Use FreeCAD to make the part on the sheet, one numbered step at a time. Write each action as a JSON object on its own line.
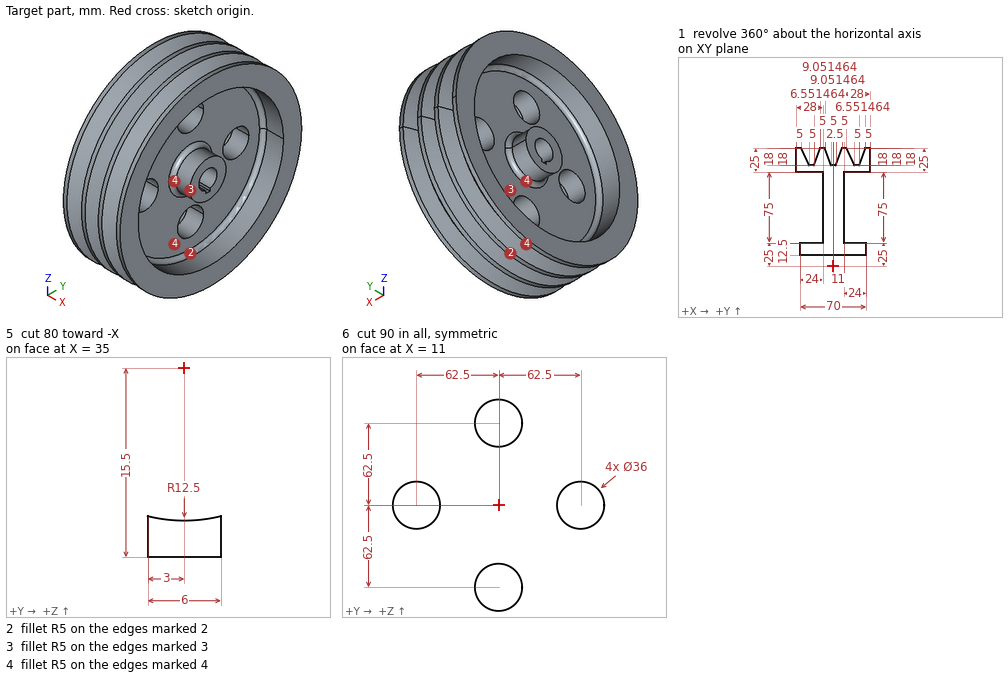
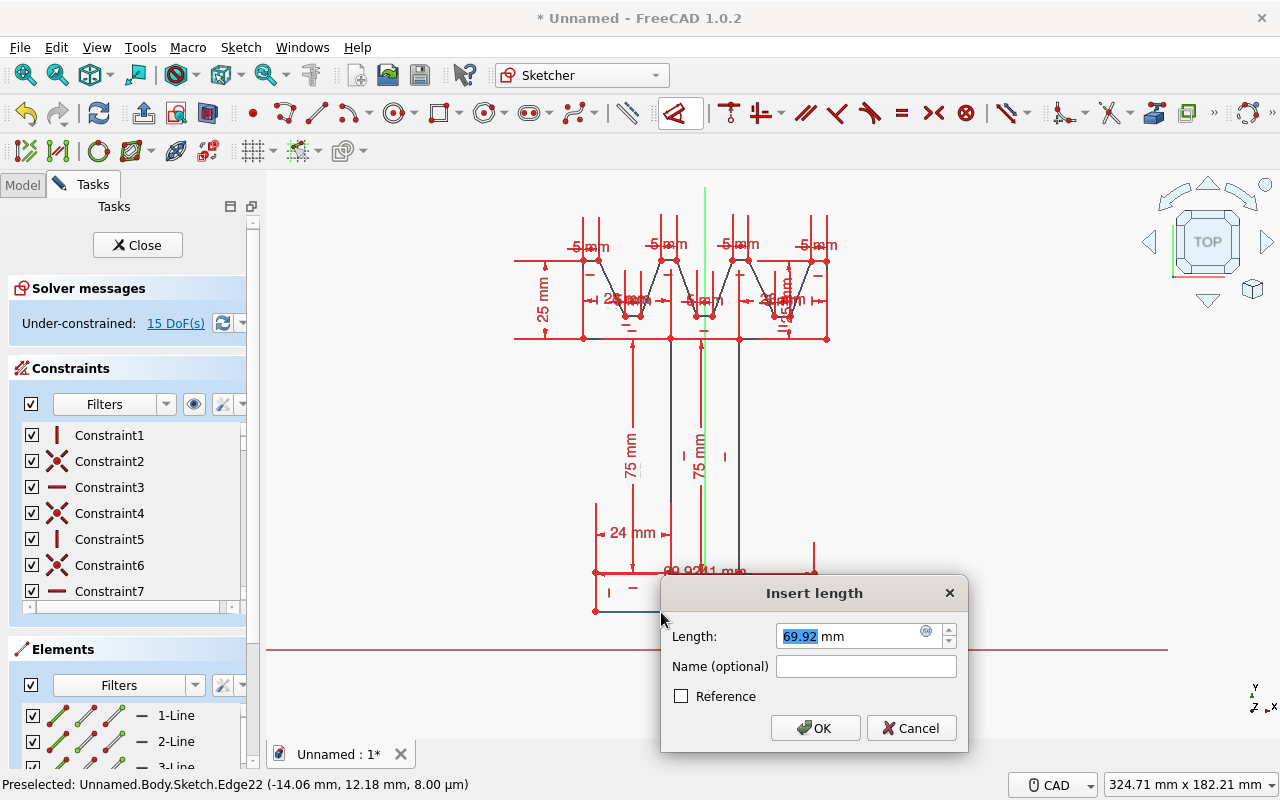
{"action": "type", "text": "70"}
{"action": "key", "text": "Return"}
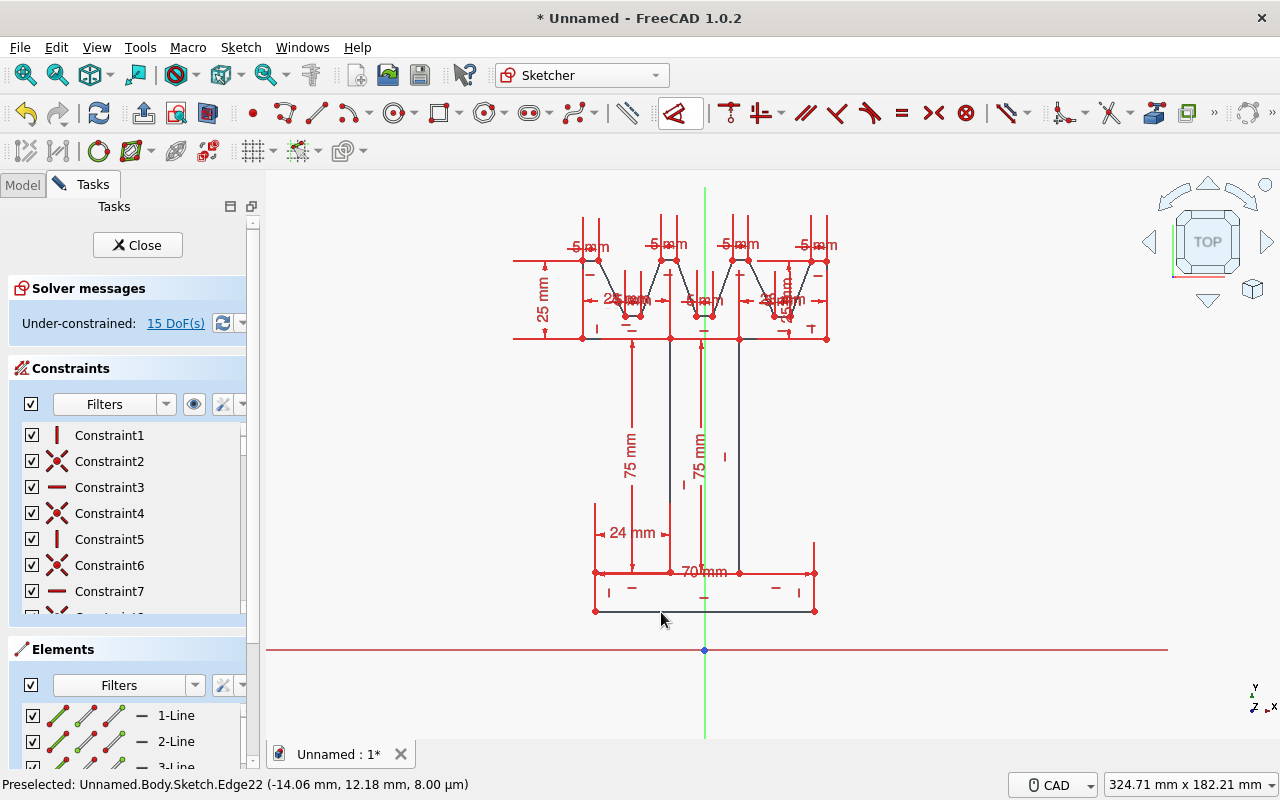
{"action": "left_click", "coordinate": [792, 573]}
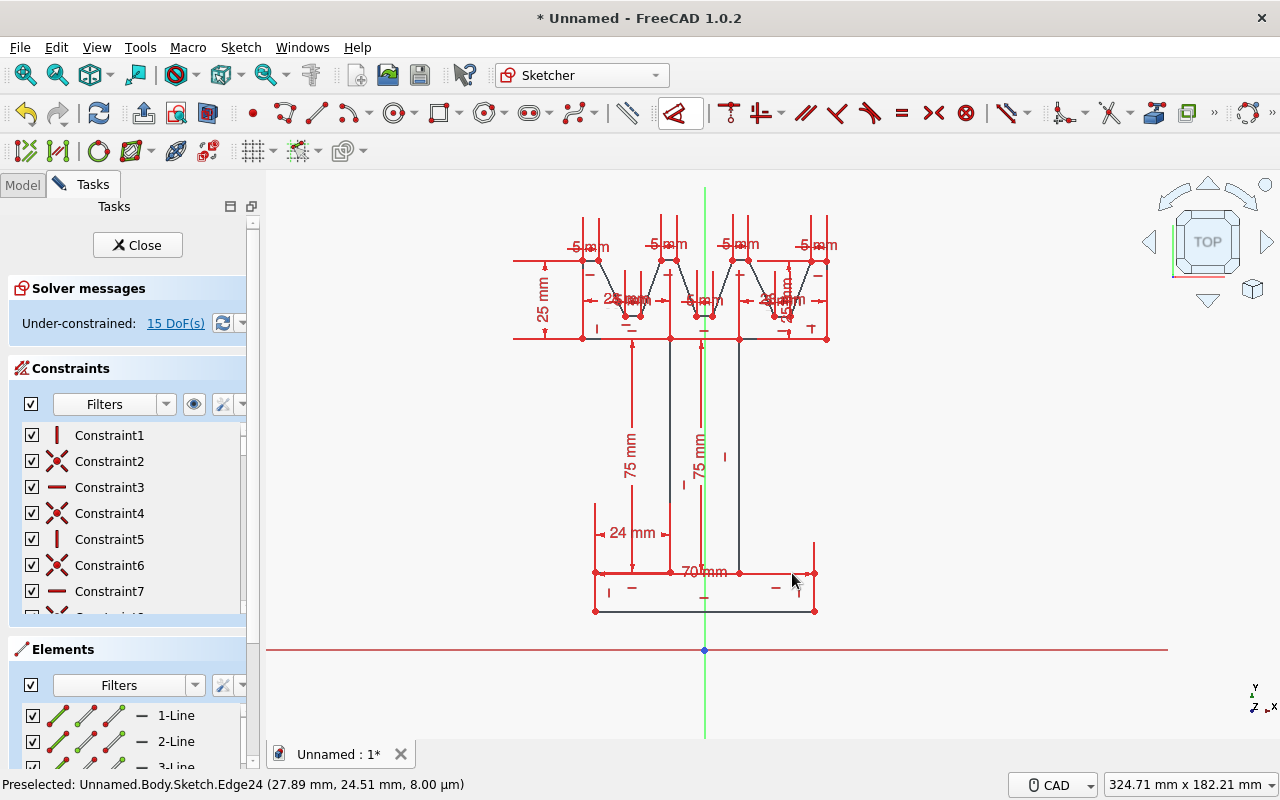
{"action": "key", "text": "l"}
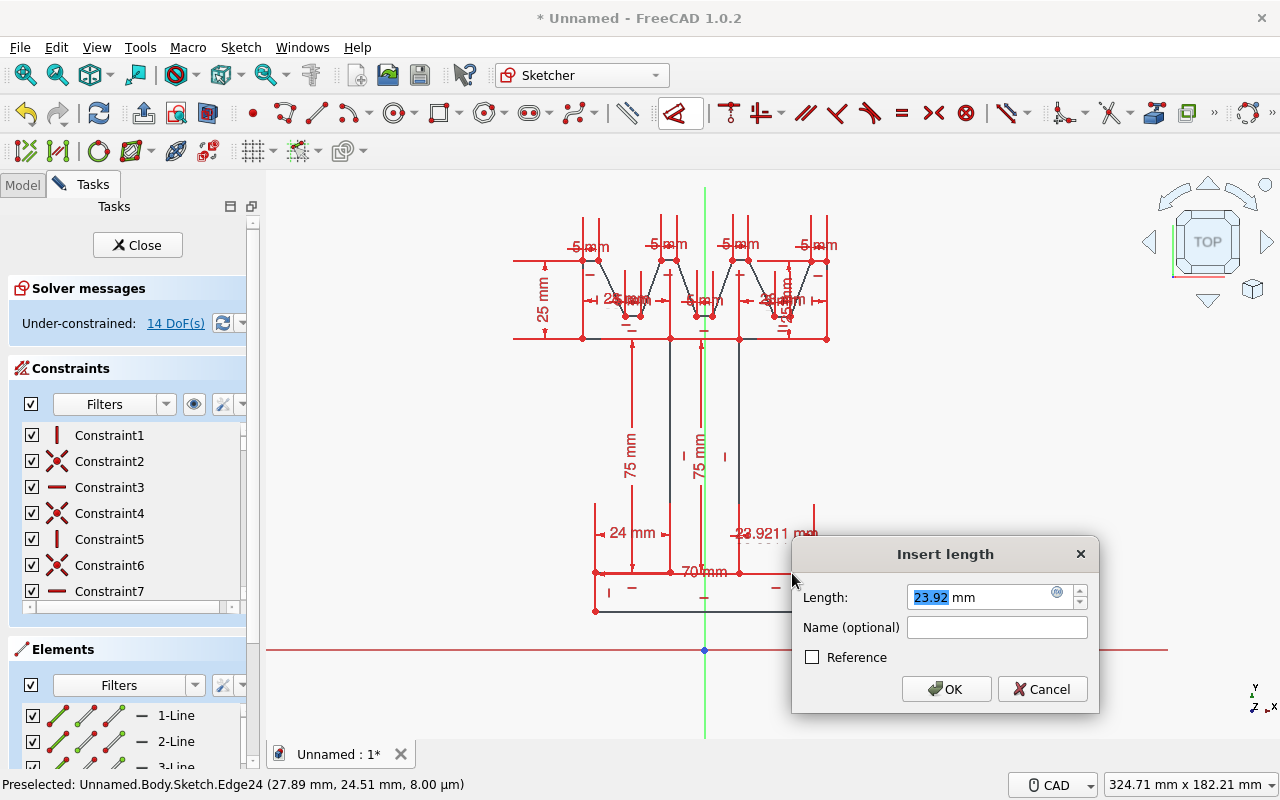
{"action": "type", "text": "24"}
{"action": "key", "text": "Return"}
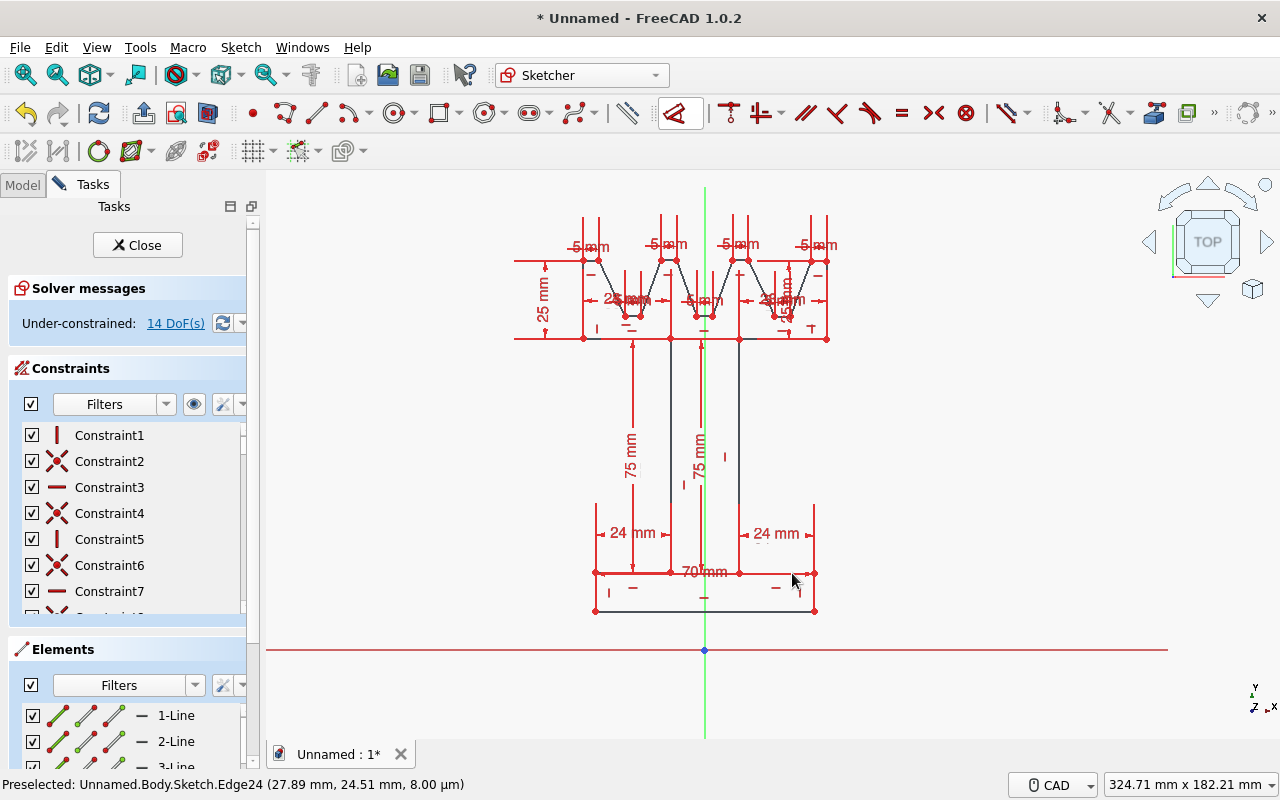
{"action": "left_click", "coordinate": [739, 573]}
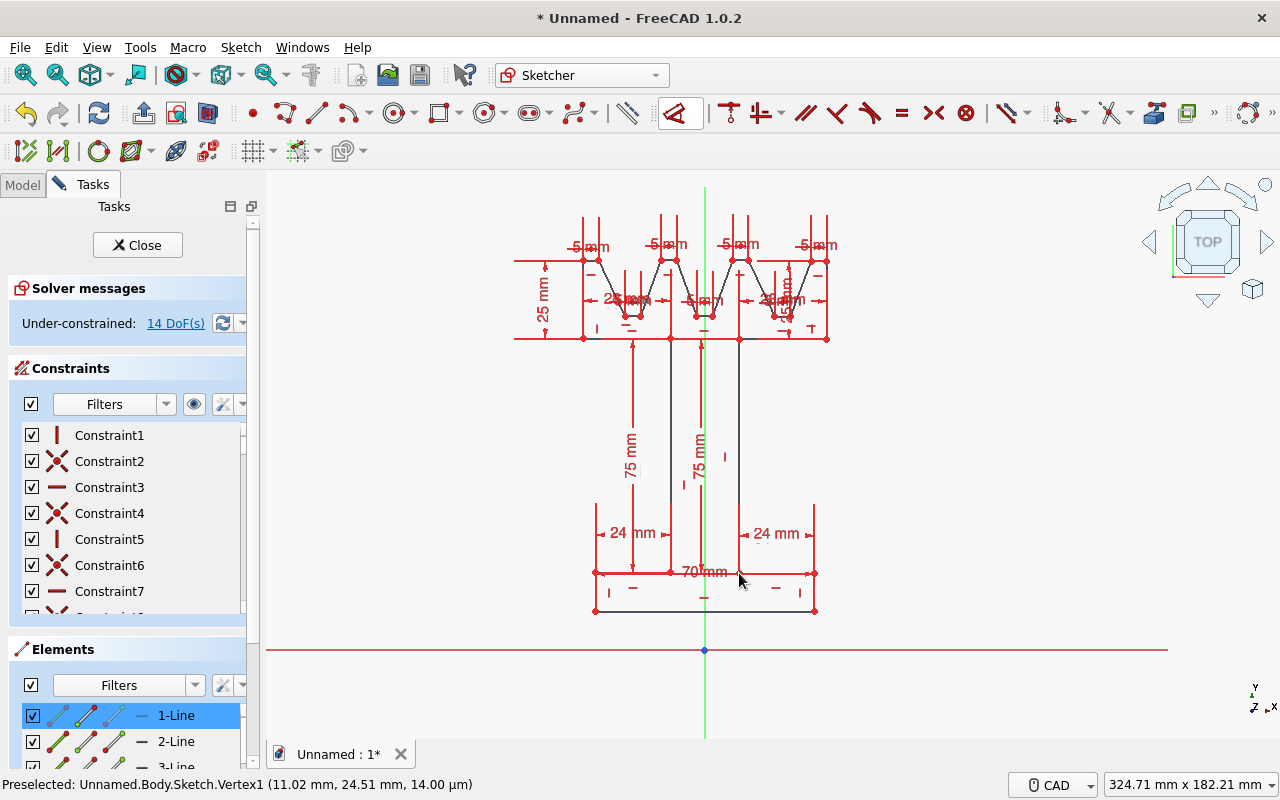
{"action": "left_click", "coordinate": [698, 114]}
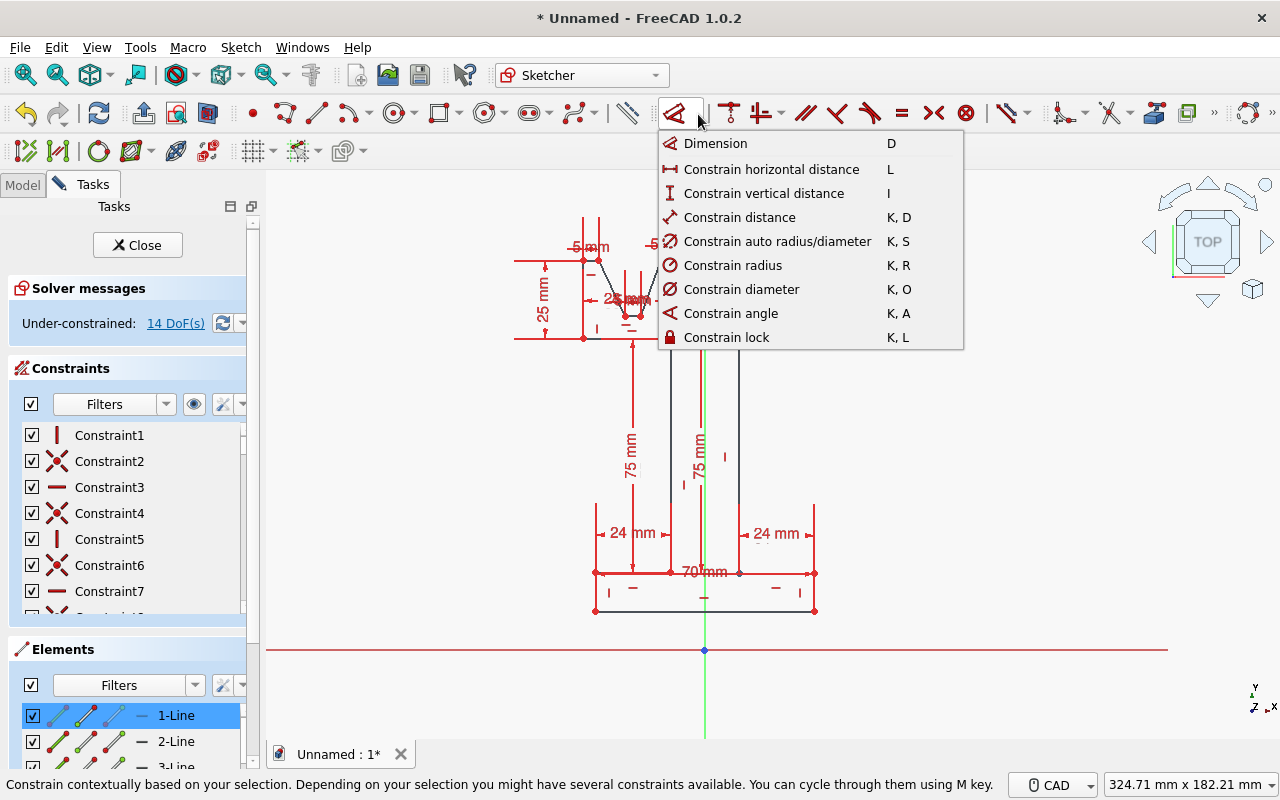
{"action": "left_click", "coordinate": [811, 169]}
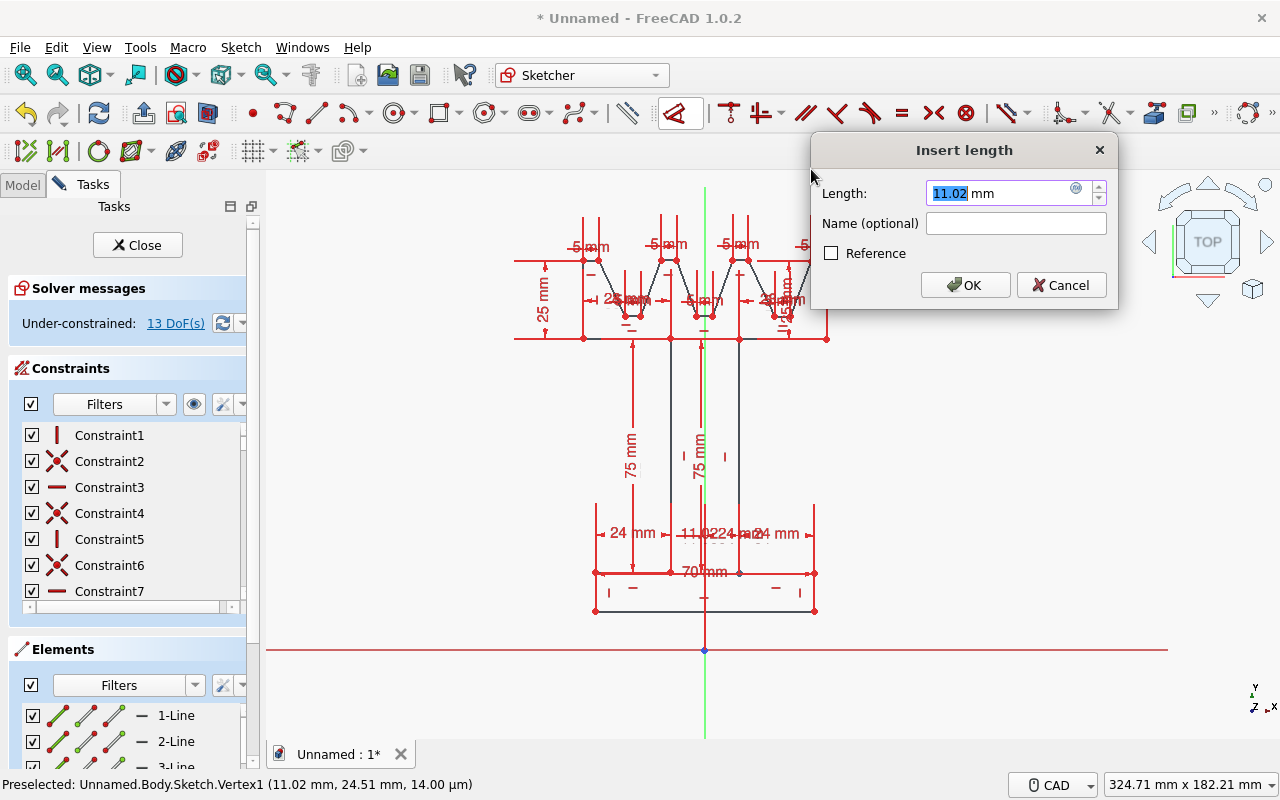
{"action": "type", "text": "11"}
{"action": "key", "text": "Return"}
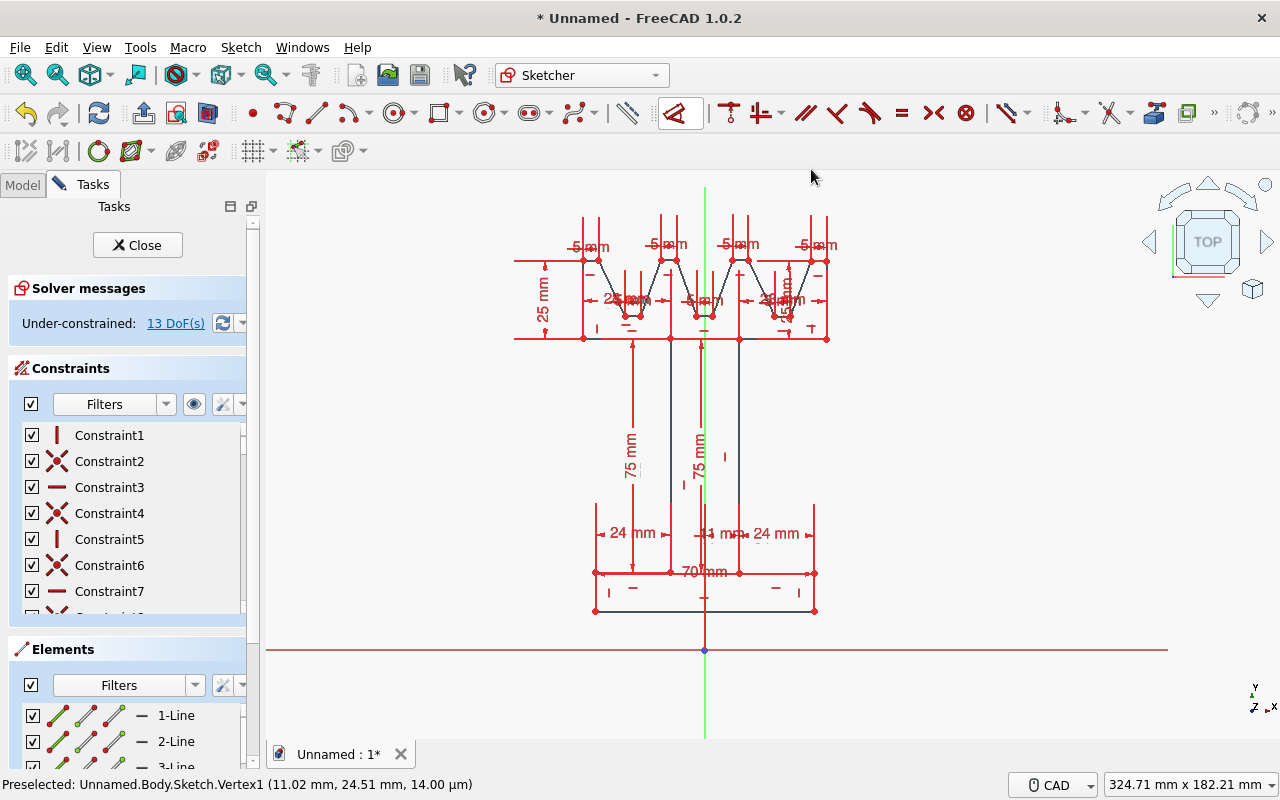
{"action": "left_click", "coordinate": [739, 573]}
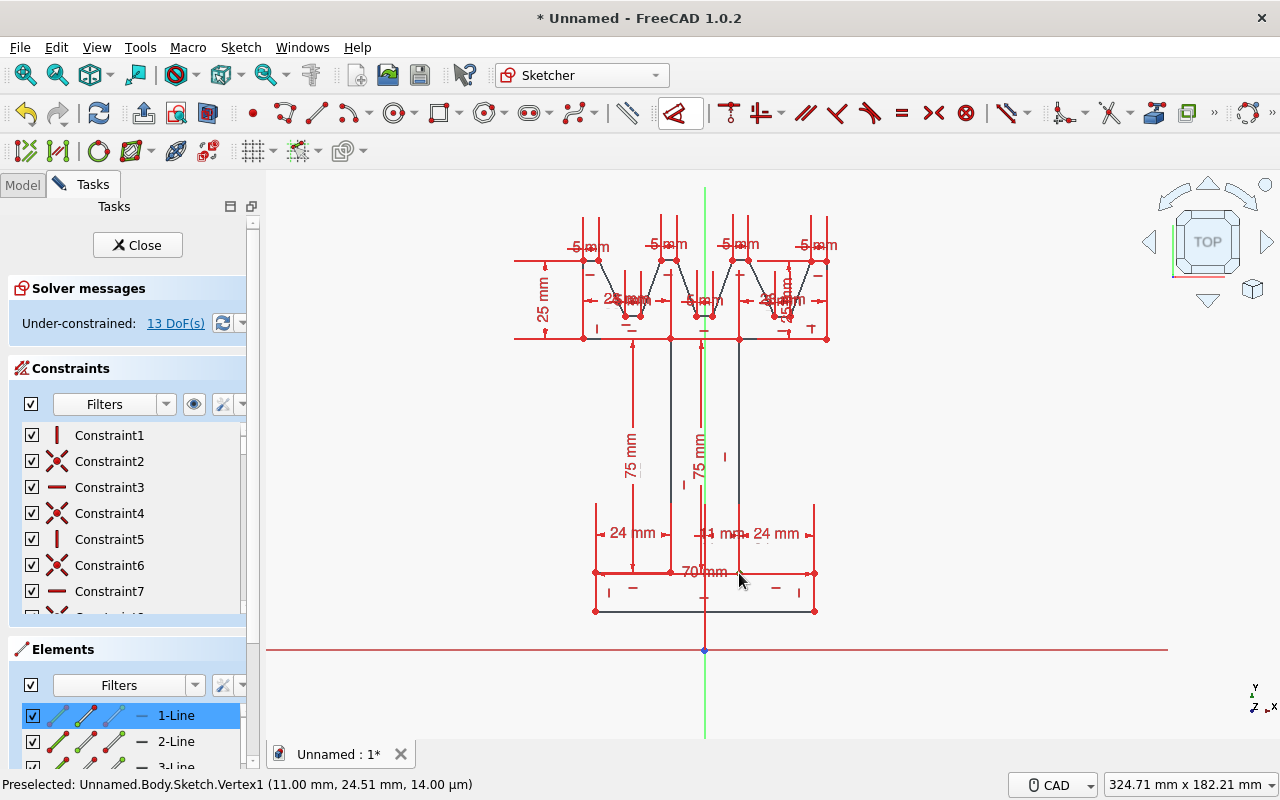
{"action": "key", "text": "i"}